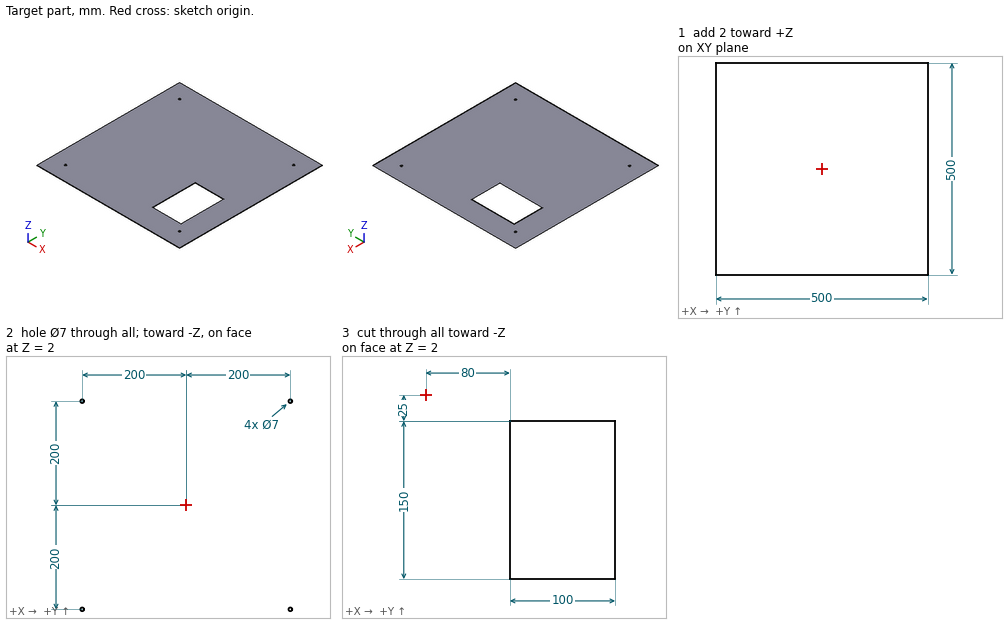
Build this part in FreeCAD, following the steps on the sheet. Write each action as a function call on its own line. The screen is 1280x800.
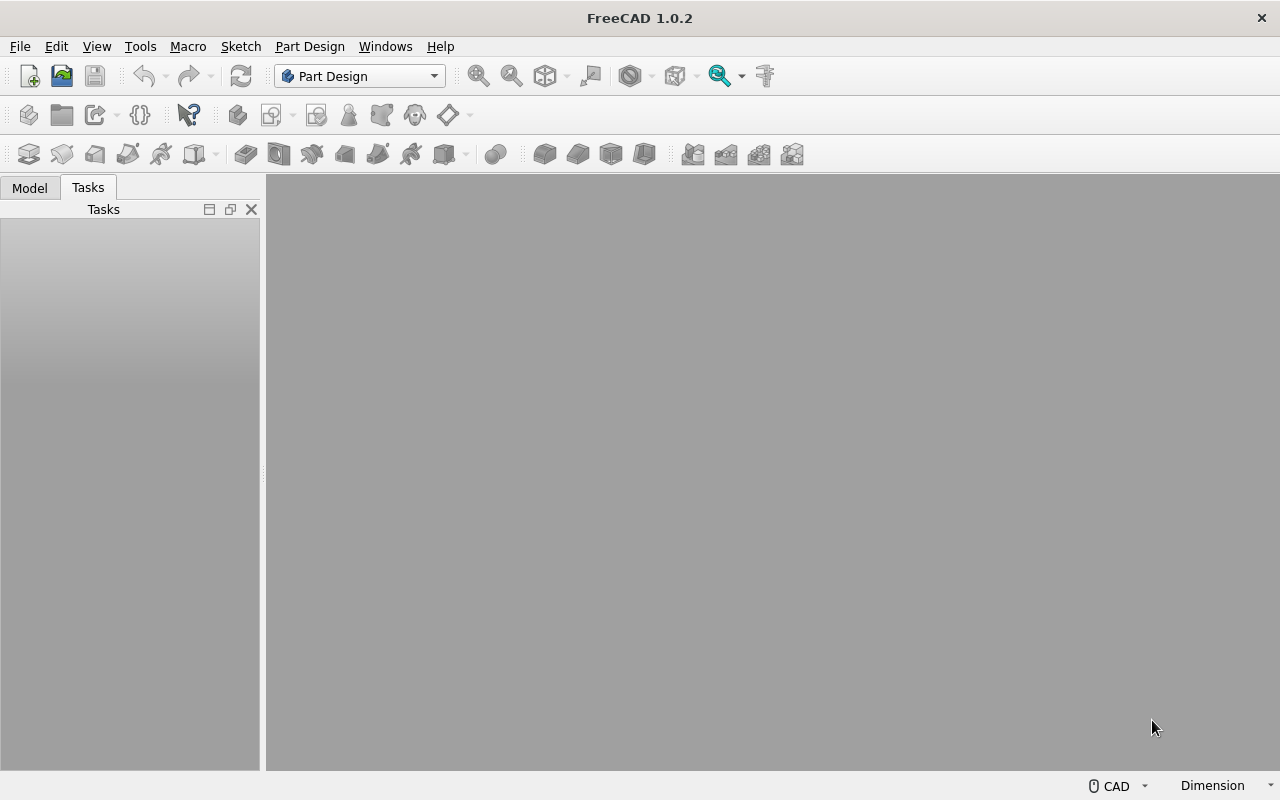
click(29, 76)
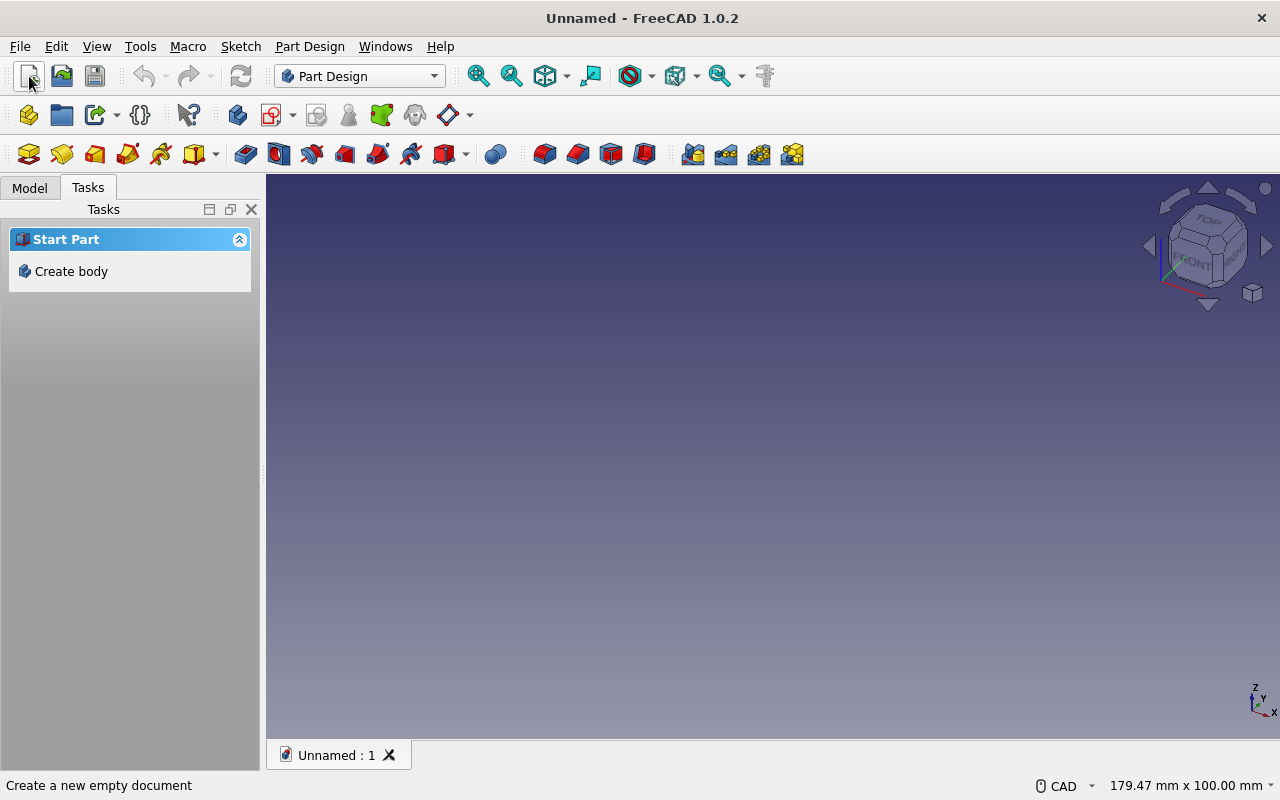
click(270, 116)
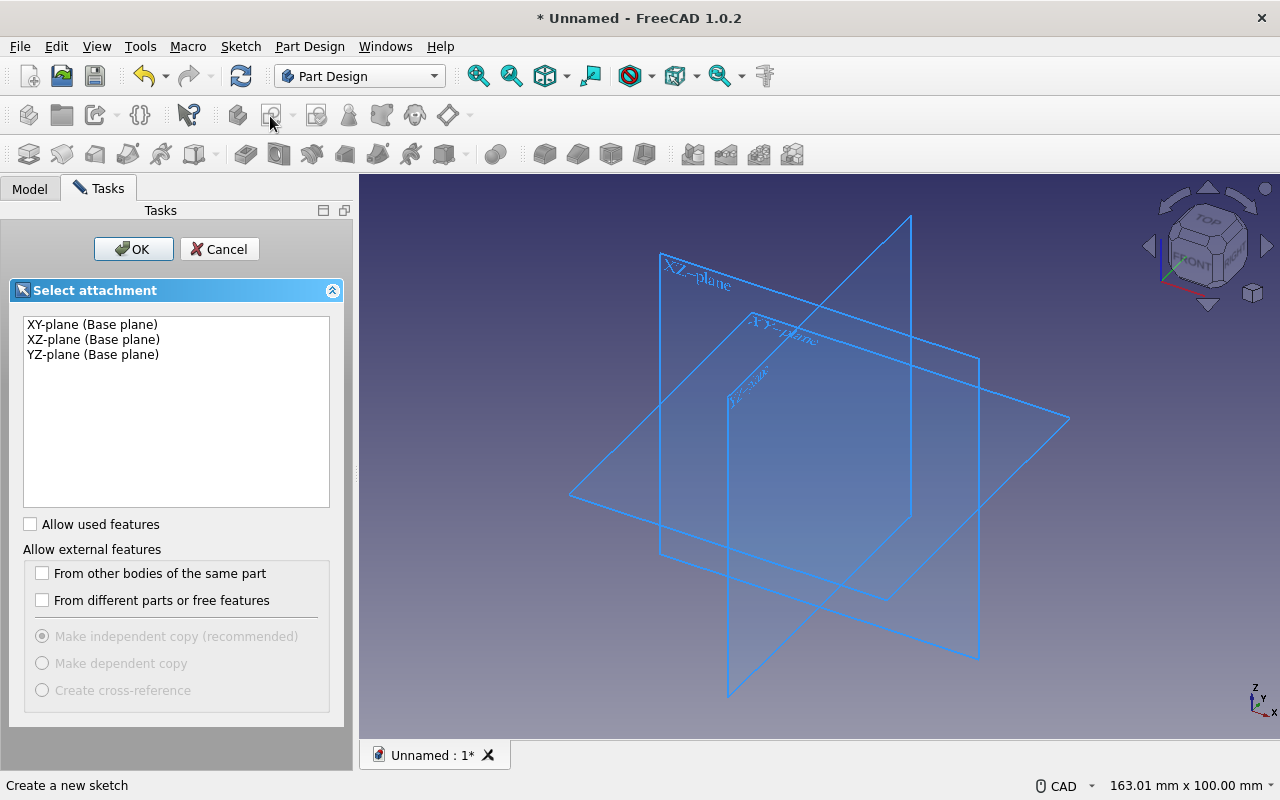
click(84, 324)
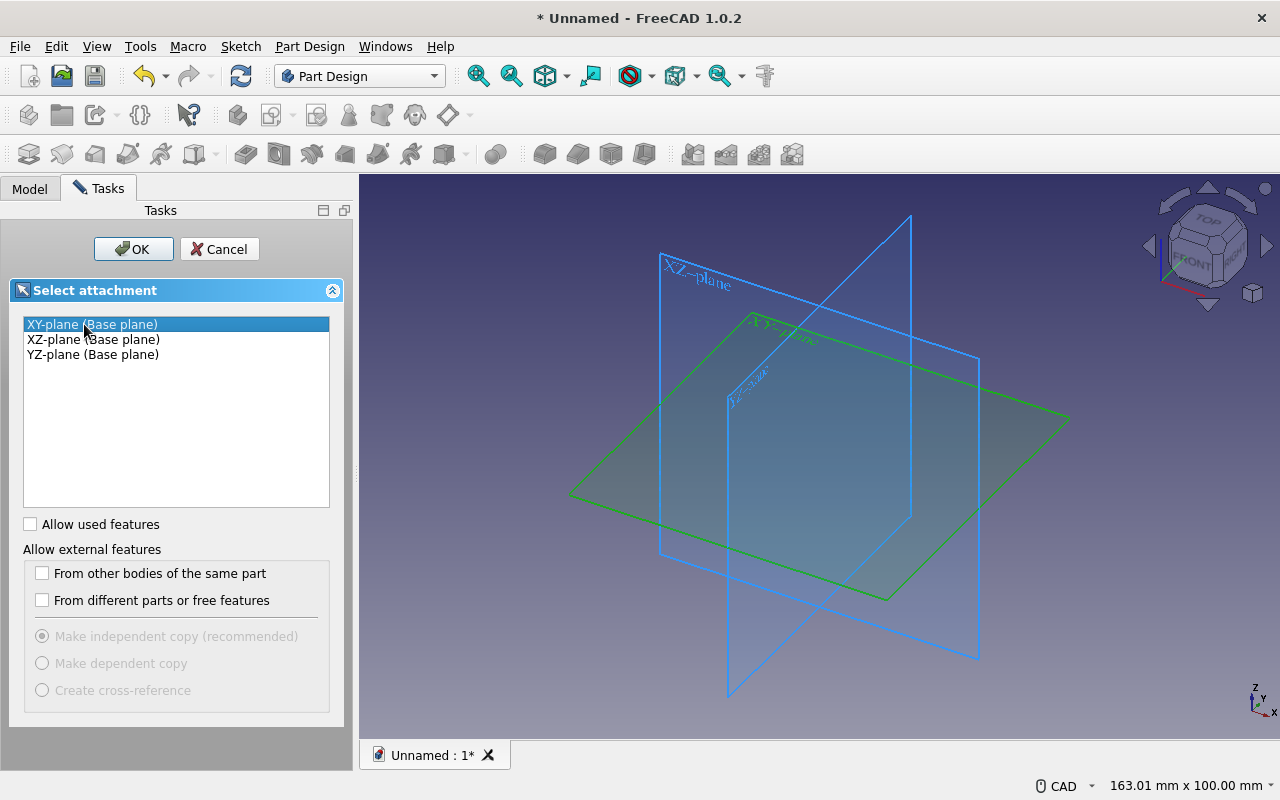
click(134, 249)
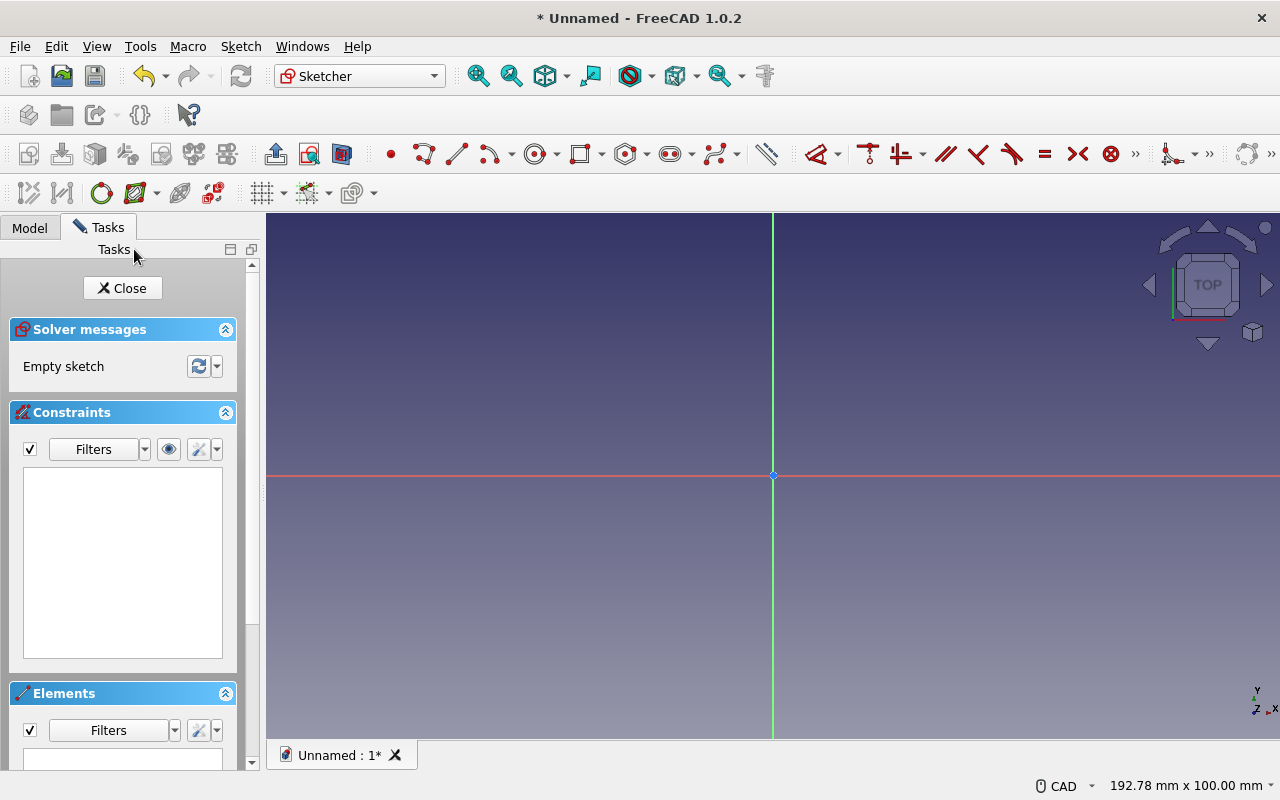
scroll(694, 476, down, 10)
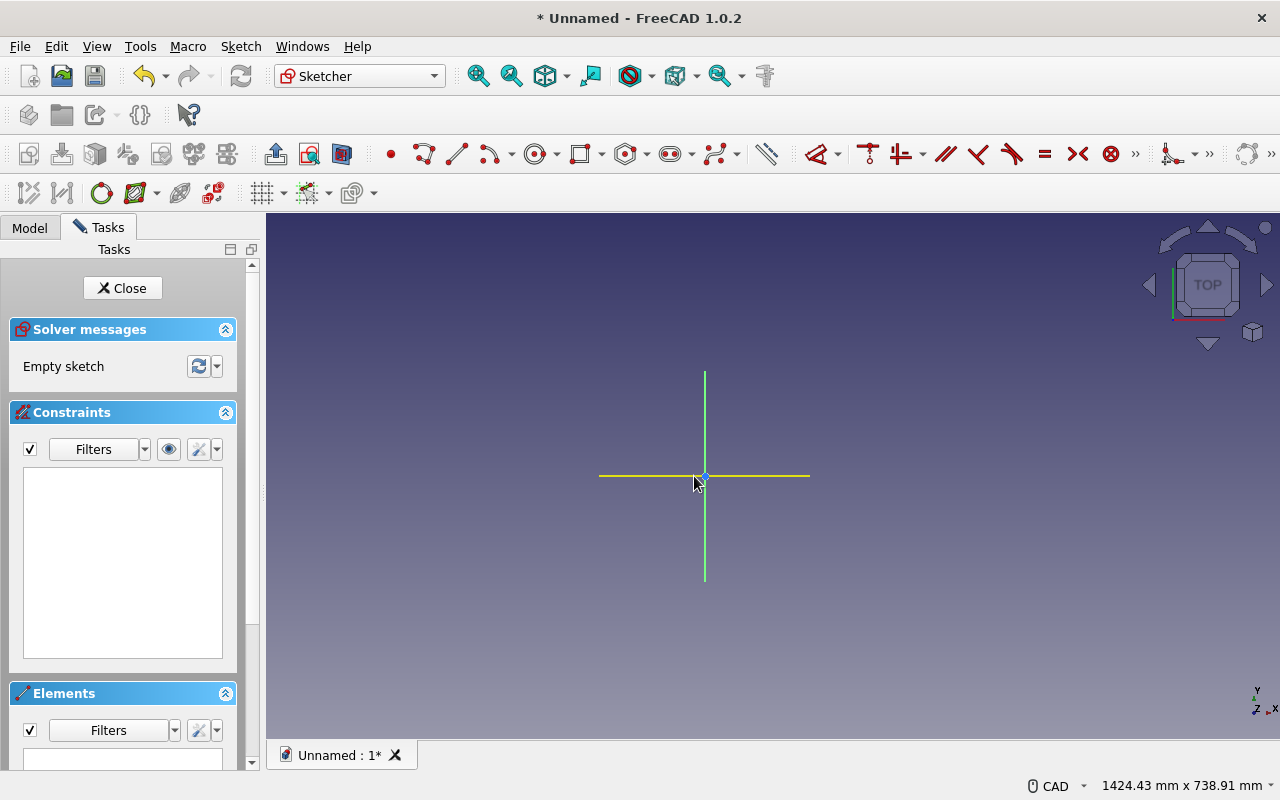
key(g)
key(v)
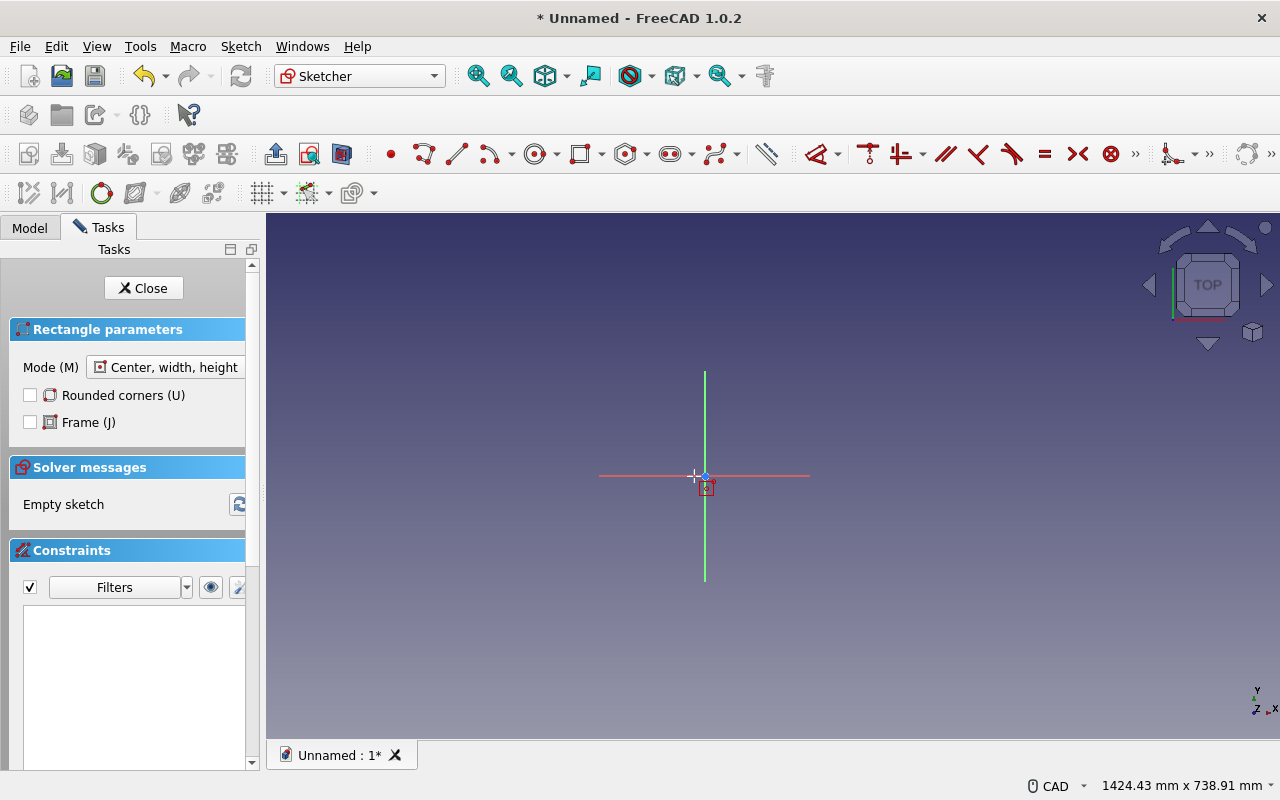
click(705, 476)
click(883, 298)
key(Escape)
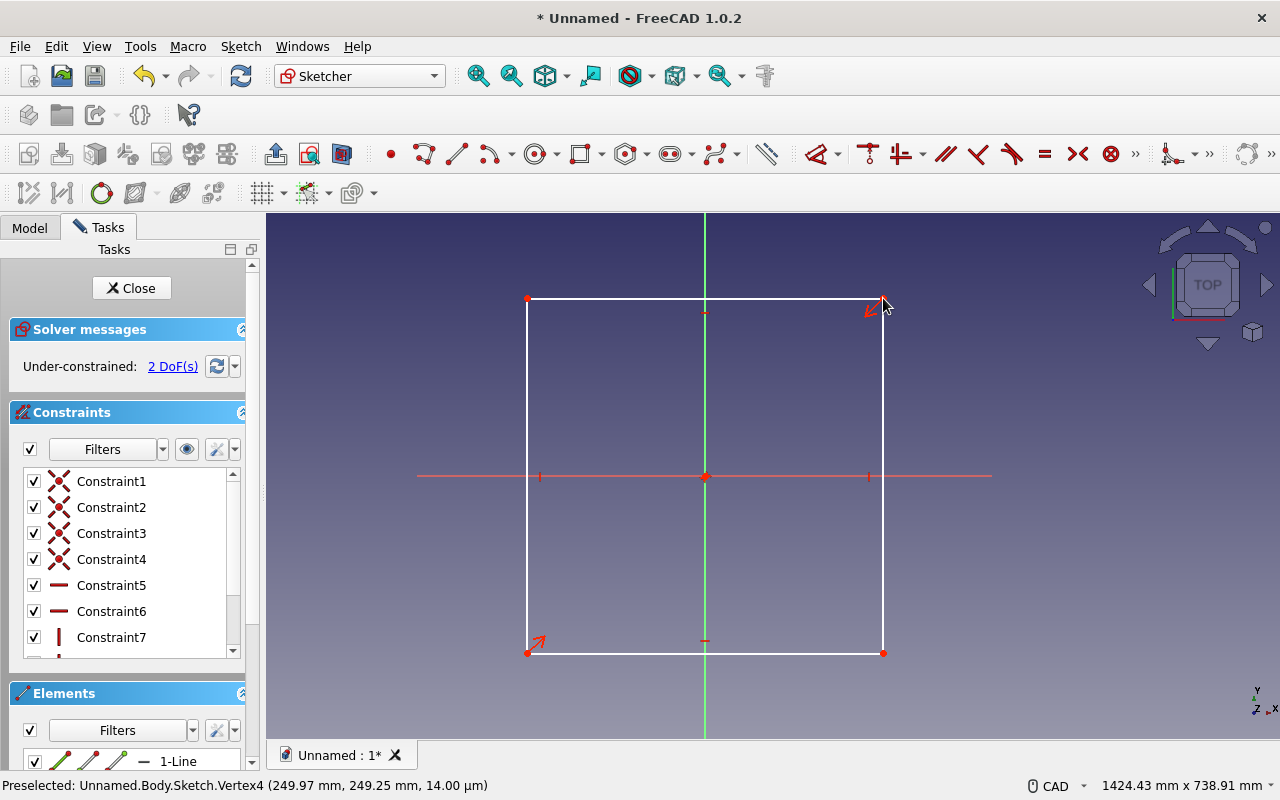
click(634, 654)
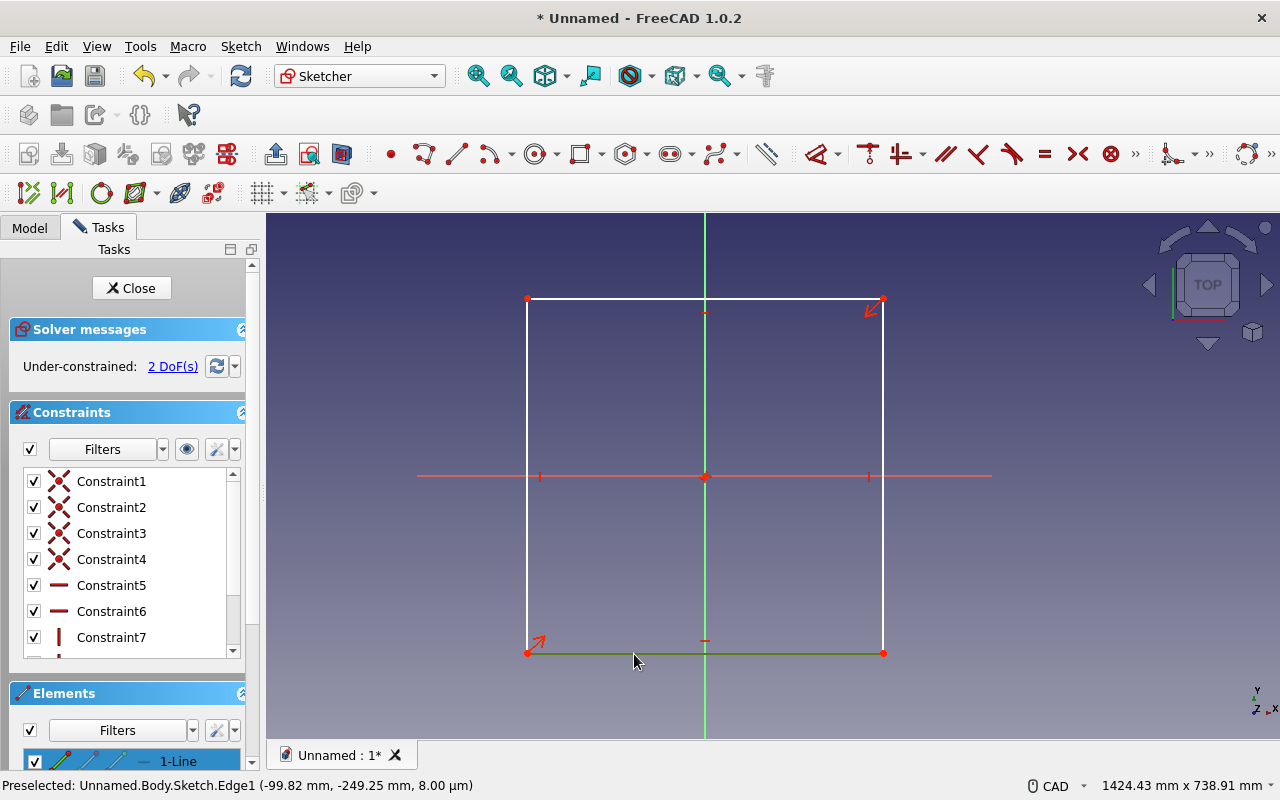
key(l)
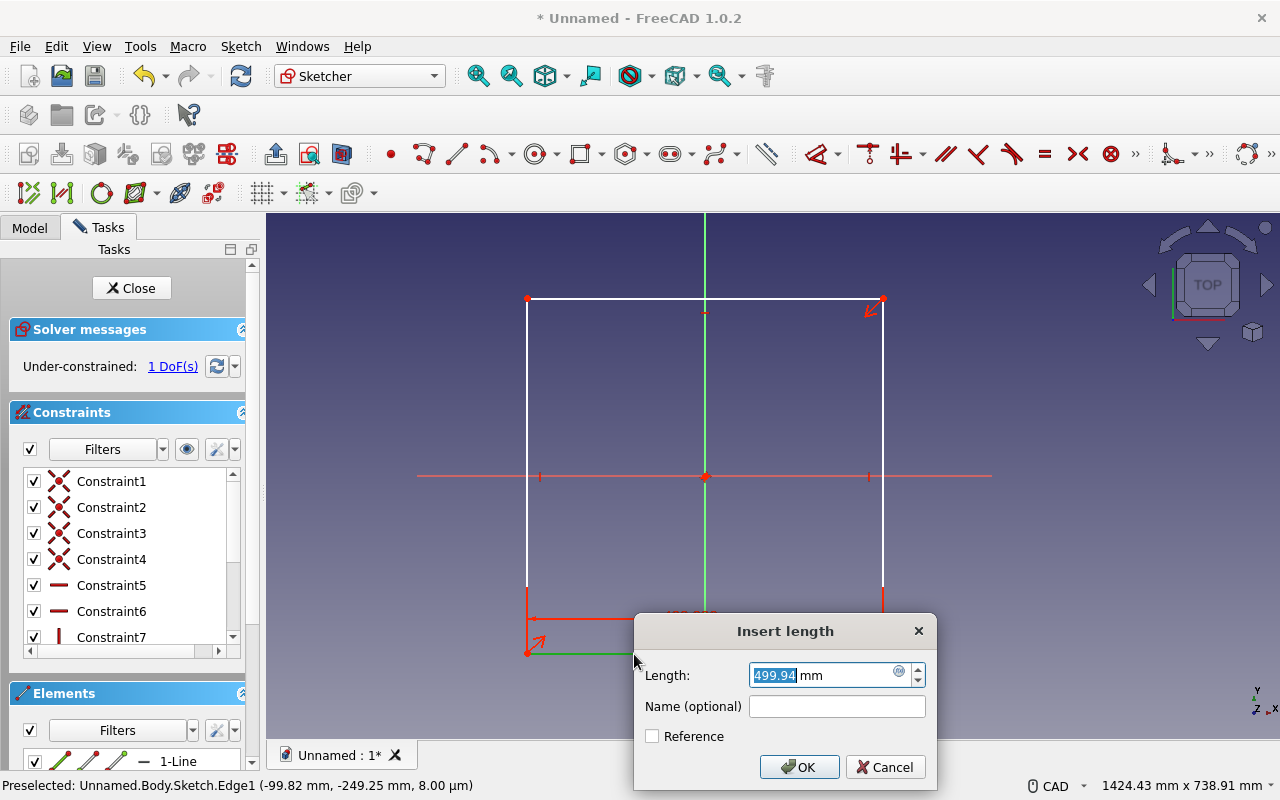
text(500)
key(Return)